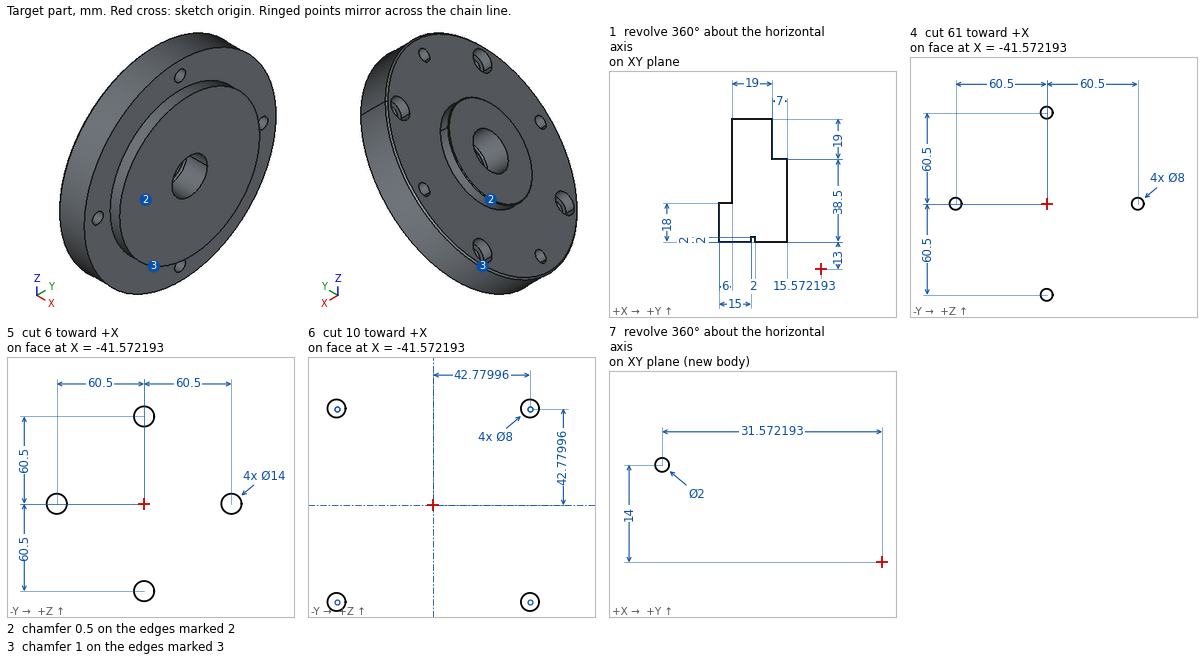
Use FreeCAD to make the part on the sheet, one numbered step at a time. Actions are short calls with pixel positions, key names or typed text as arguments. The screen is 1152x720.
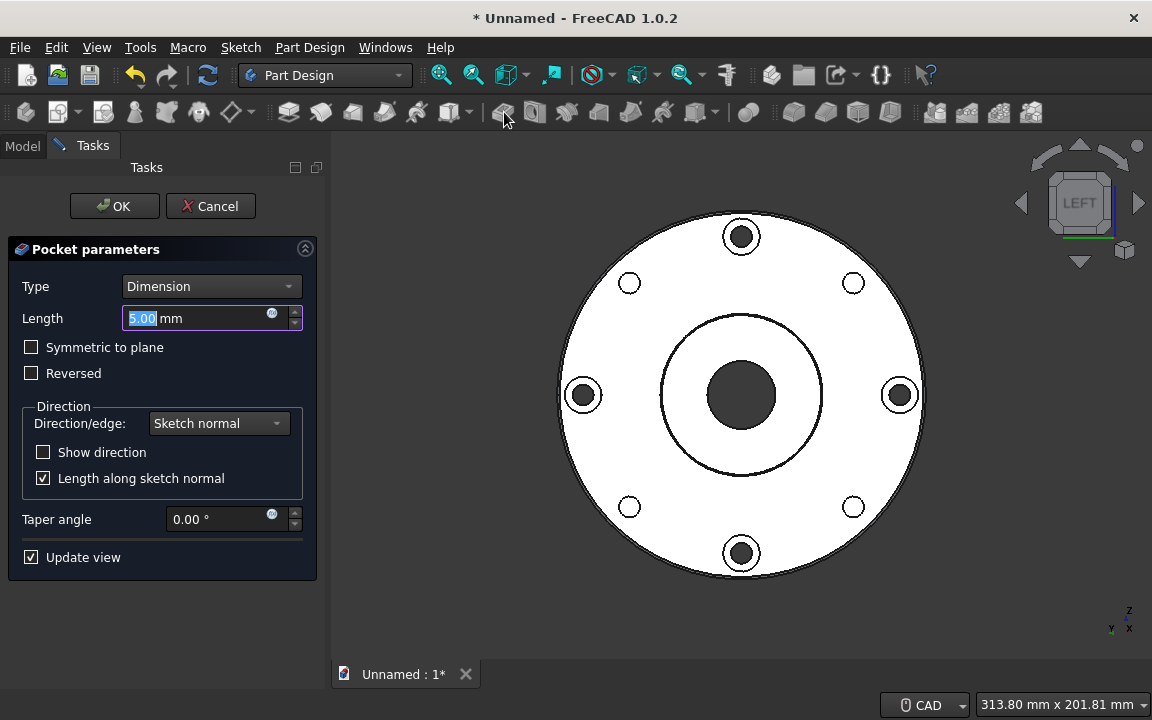
text(10)
key(Tab)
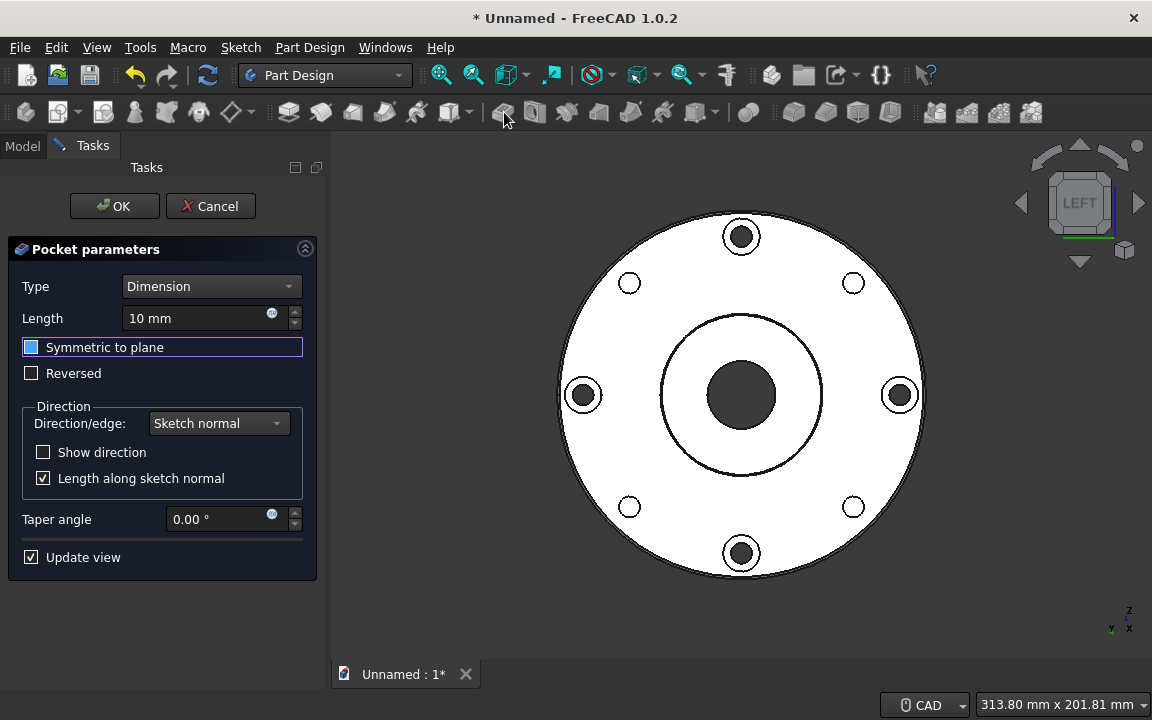
click(115, 206)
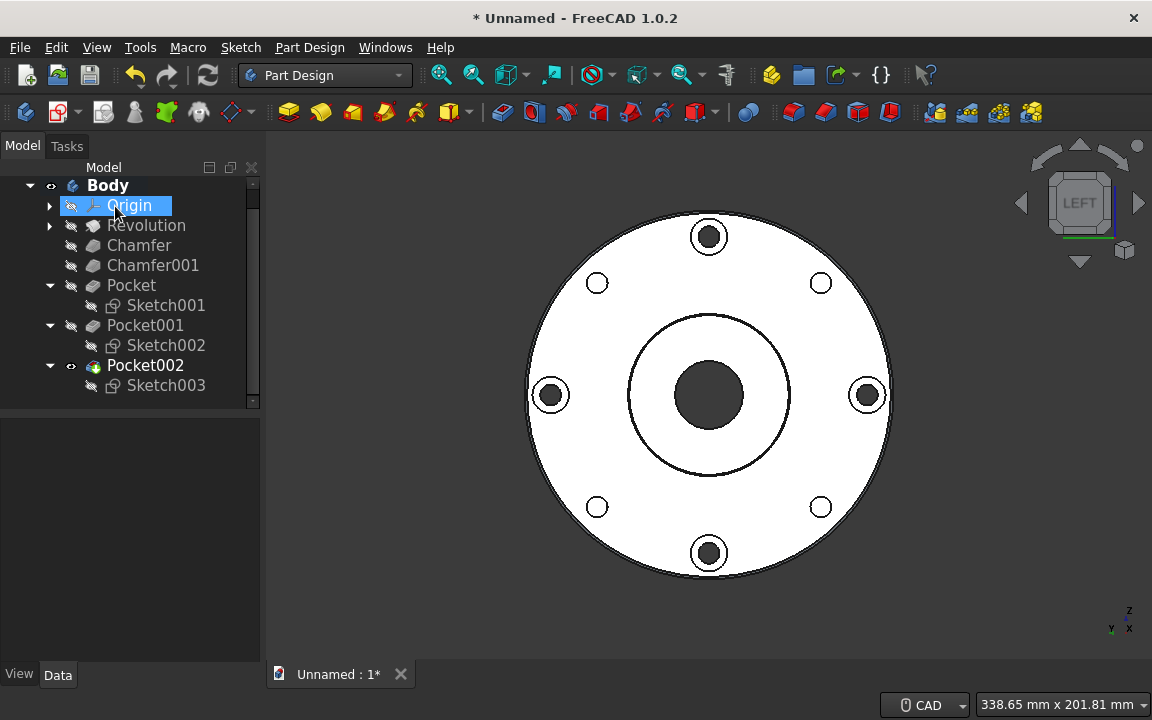
click(26, 112)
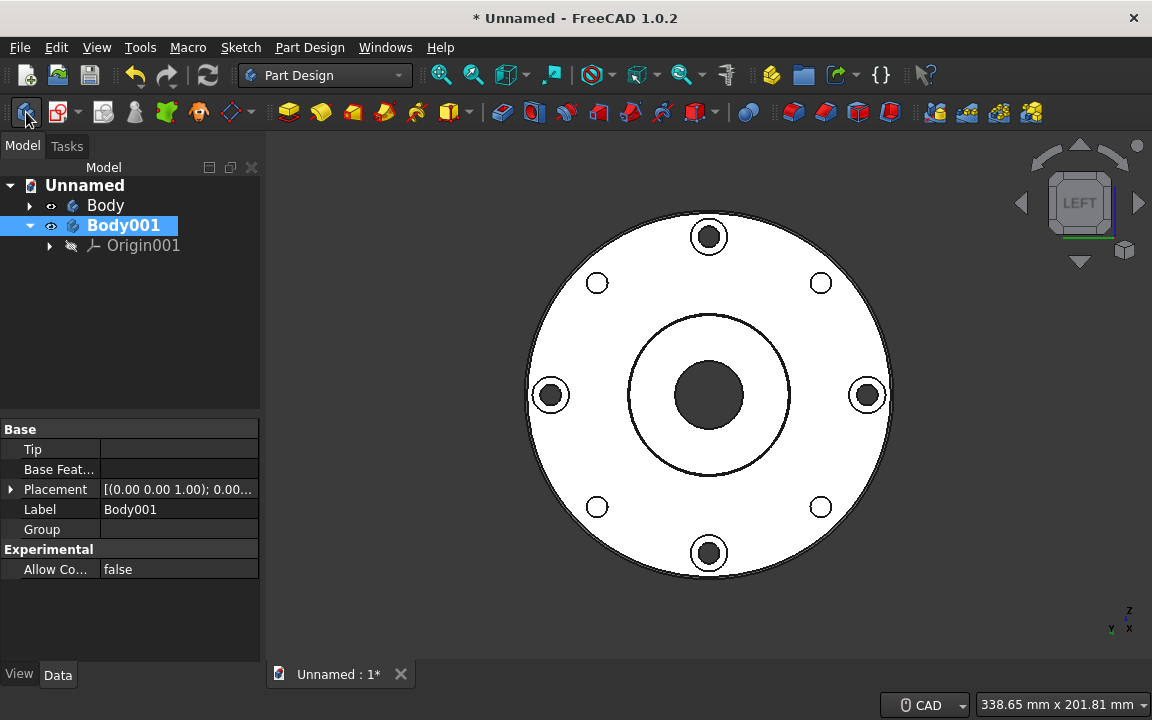
click(306, 619)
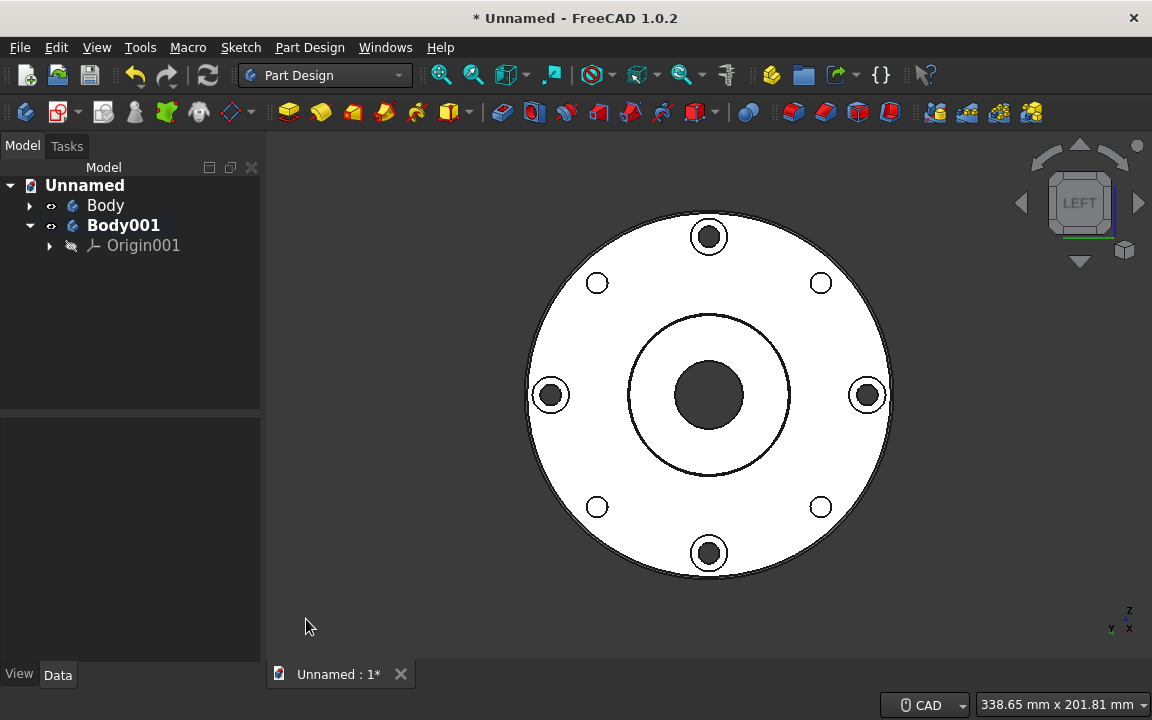
click(58, 112)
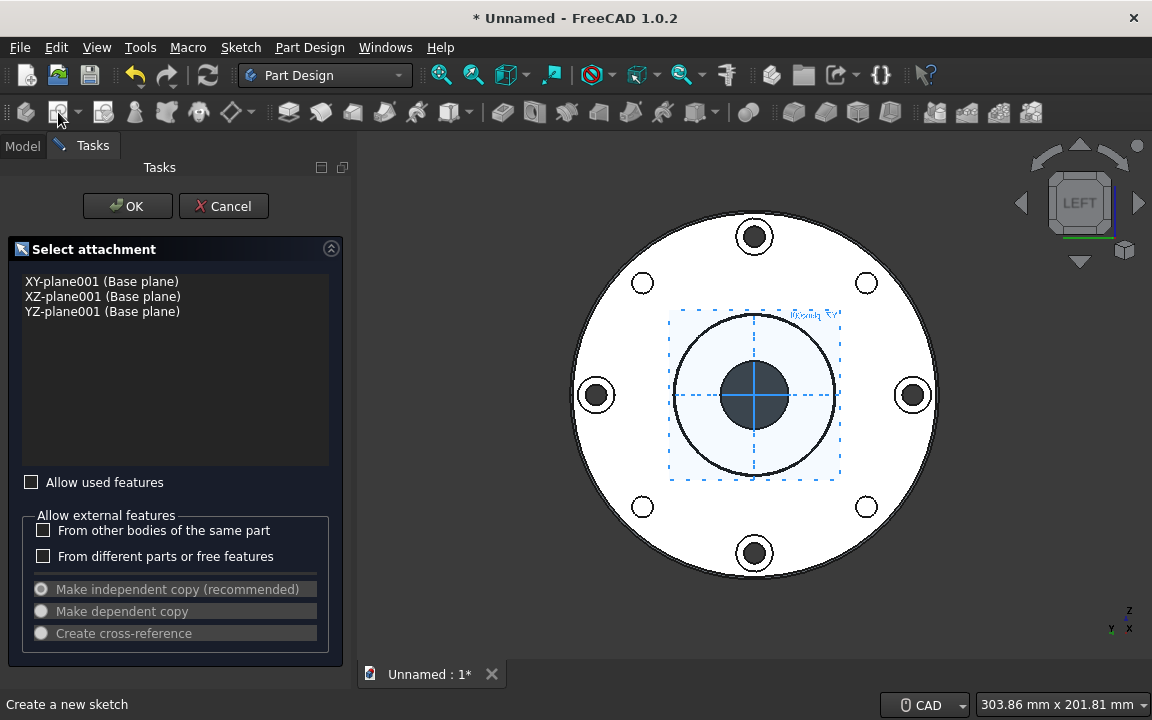
click(82, 282)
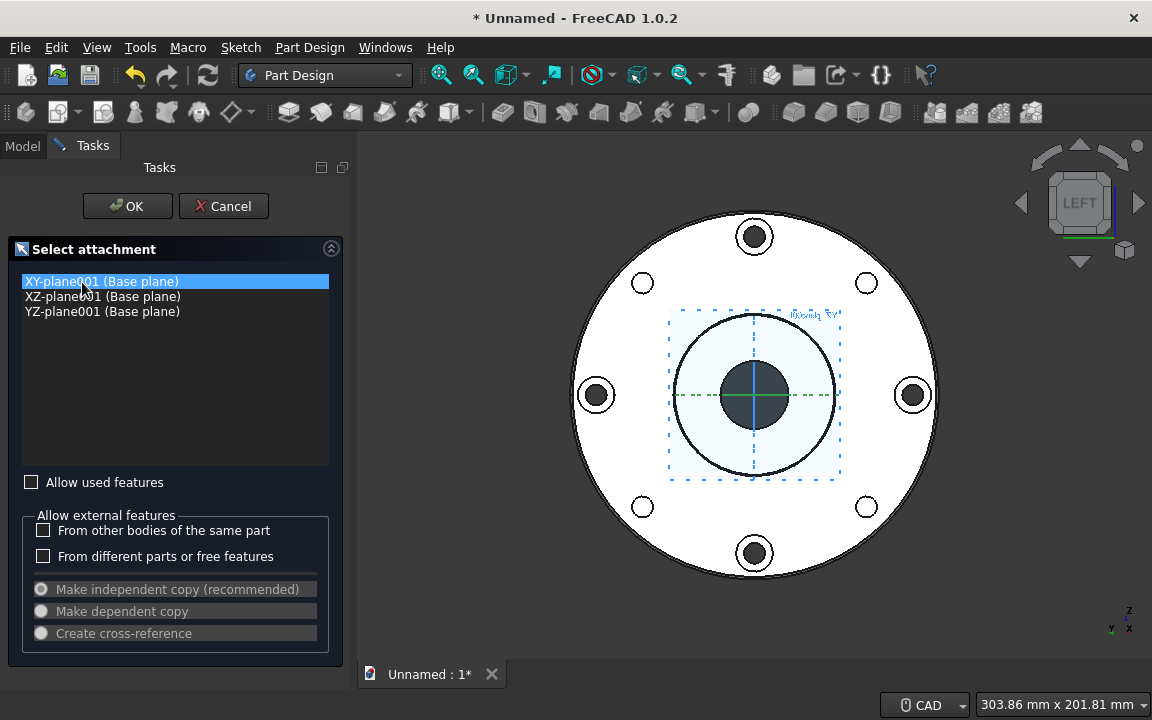
click(128, 206)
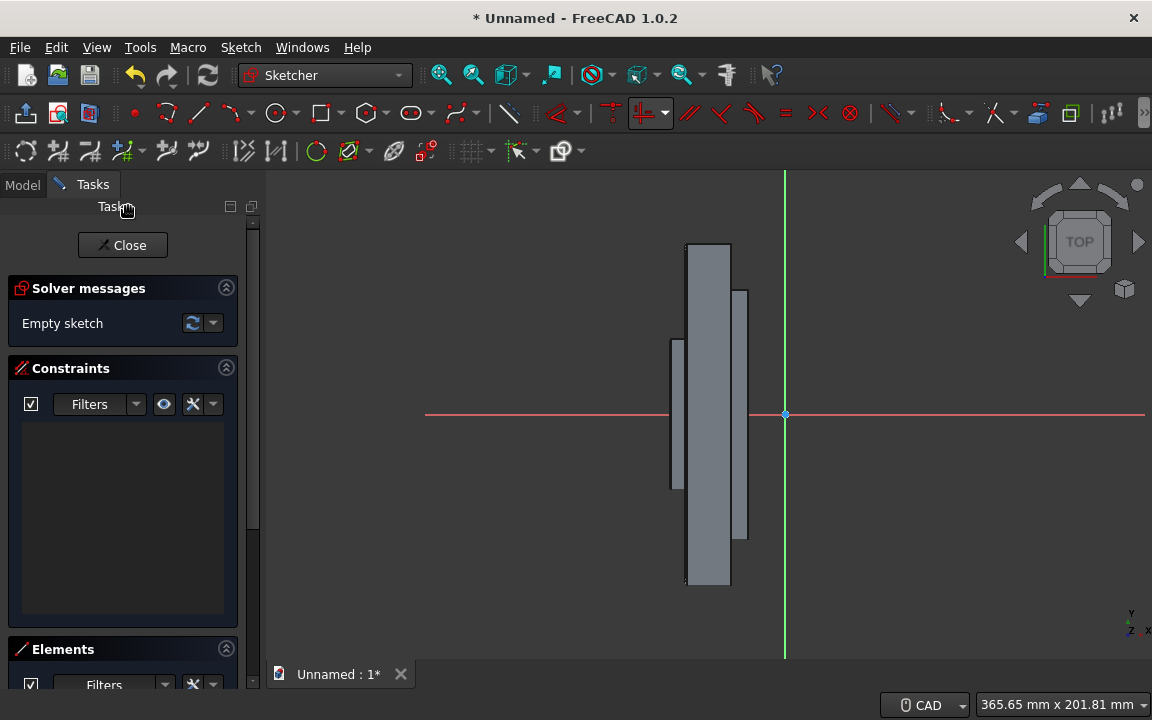
scroll(713, 379, up, 15)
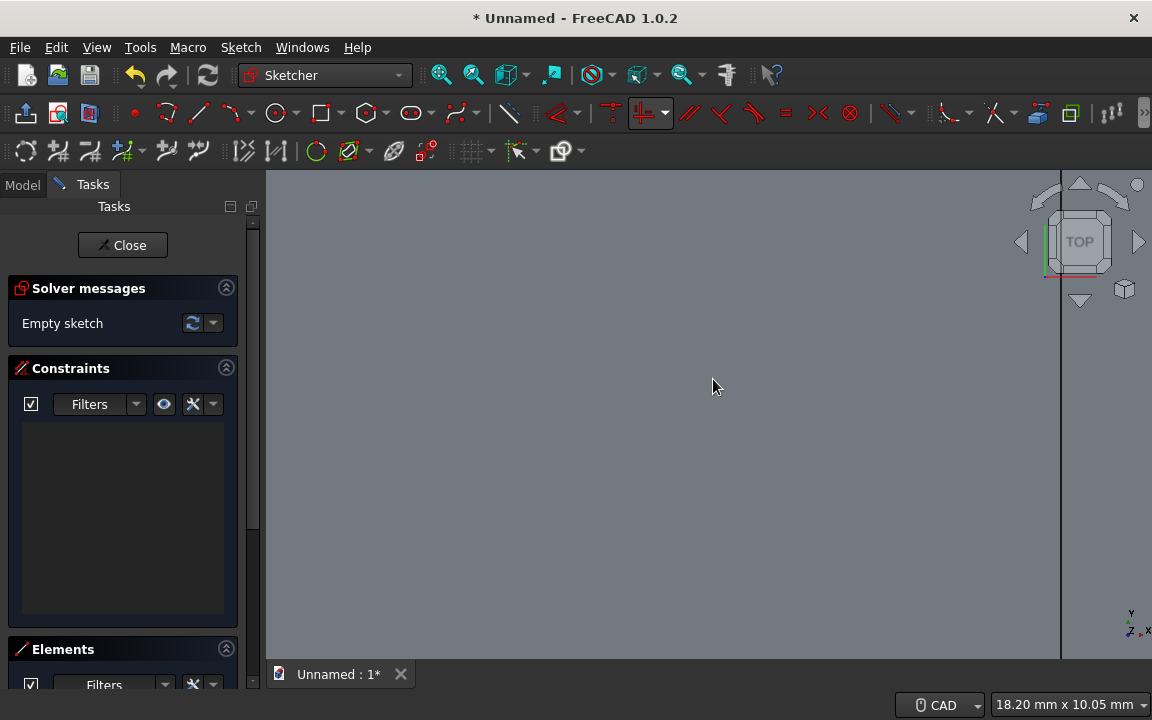
scroll(615, 397, up, 6)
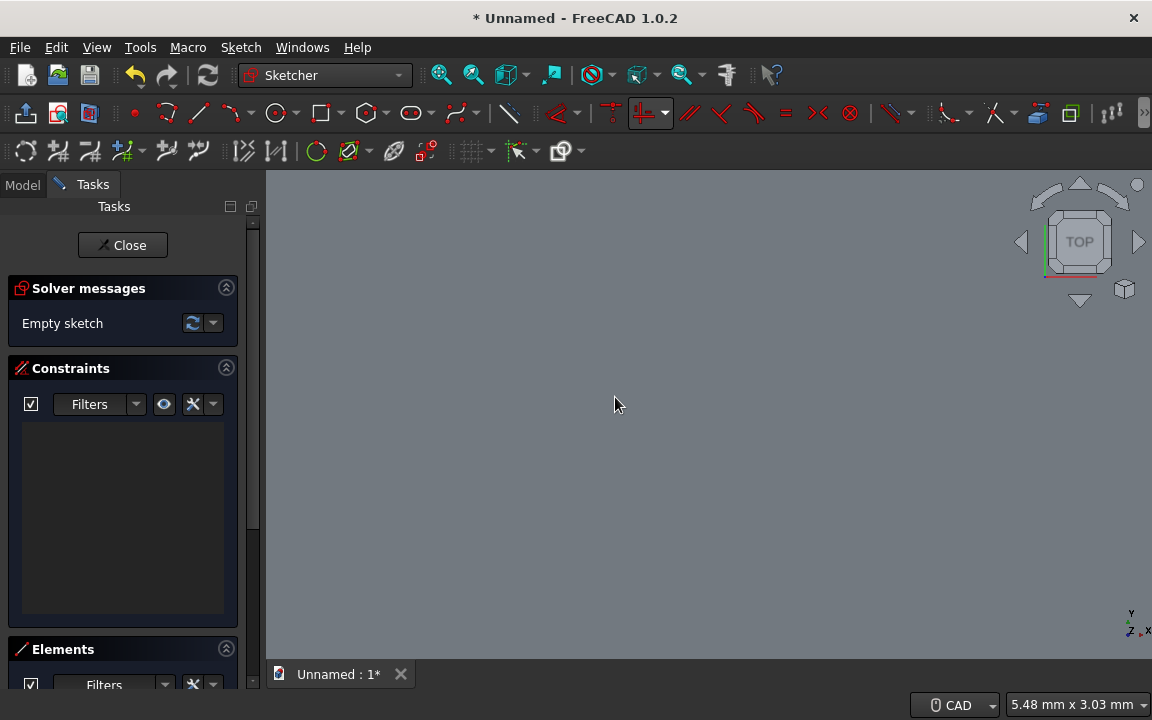
click(276, 114)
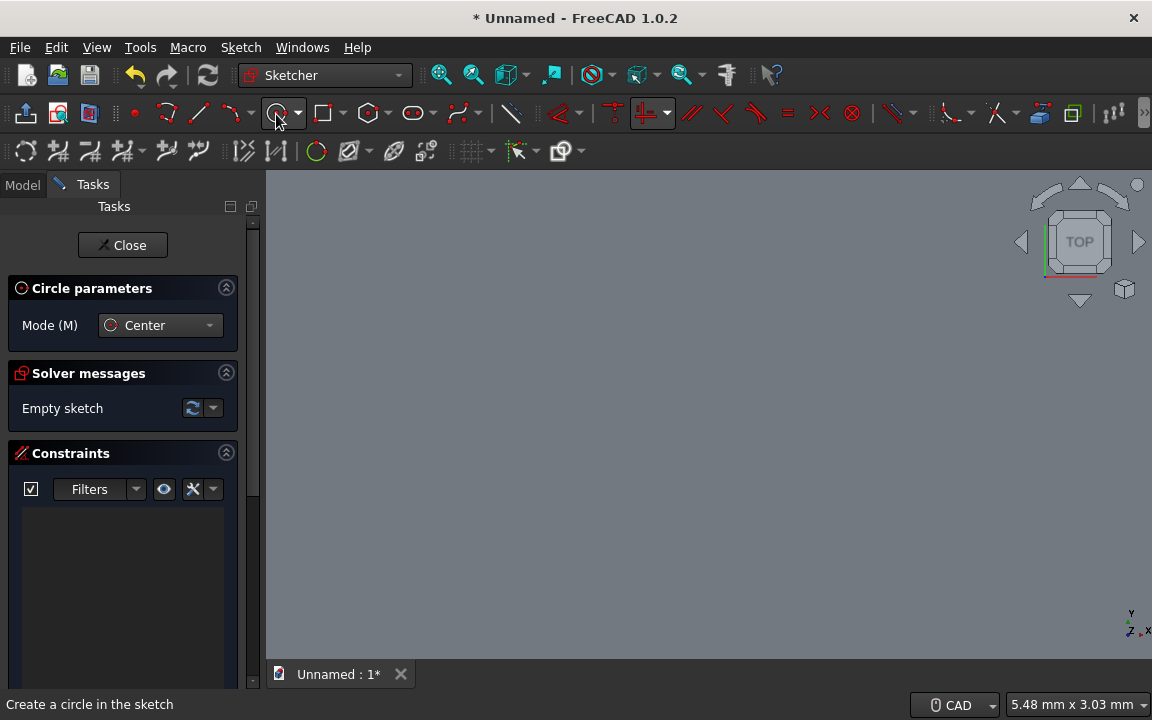
click(641, 414)
move(755, 300)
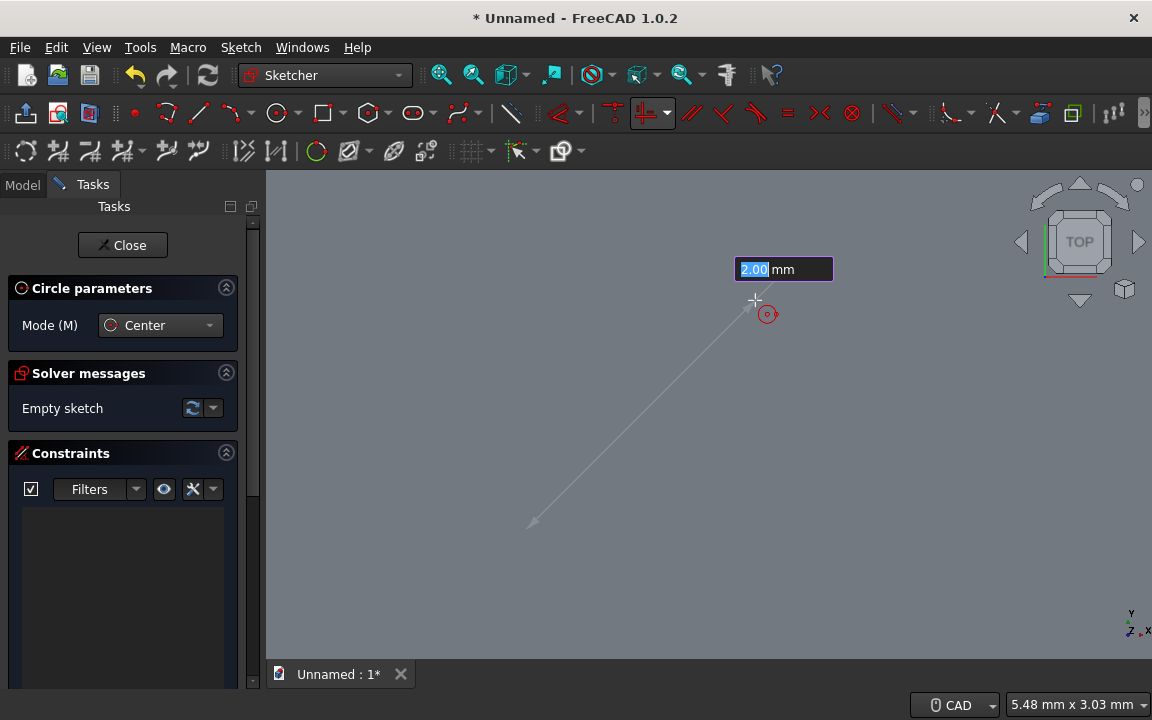
text(2)
key(Return)
key(Escape)